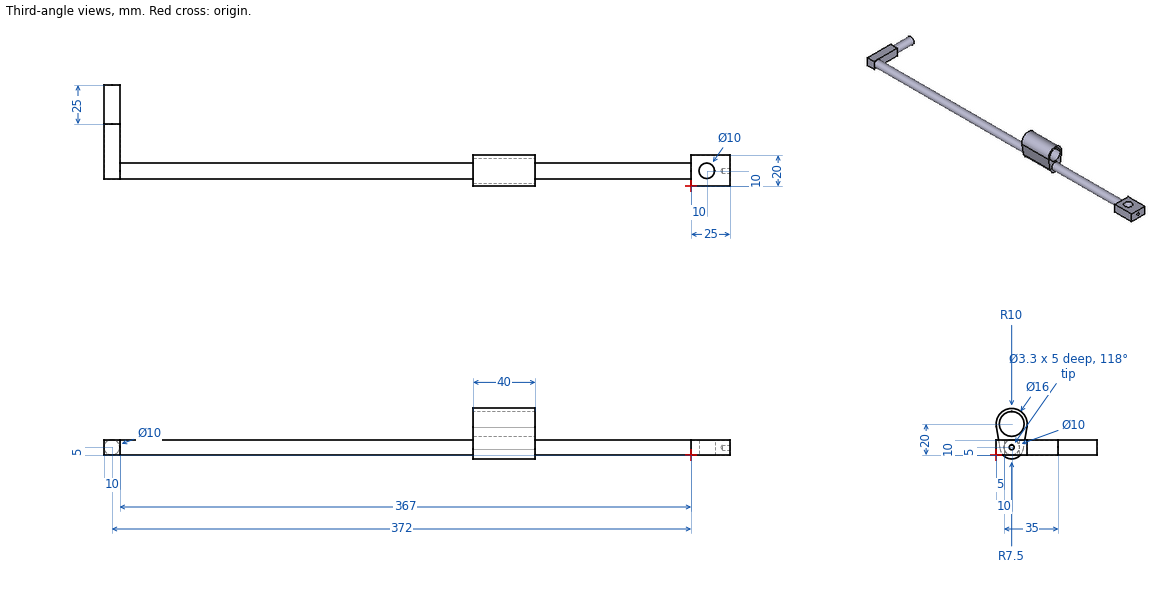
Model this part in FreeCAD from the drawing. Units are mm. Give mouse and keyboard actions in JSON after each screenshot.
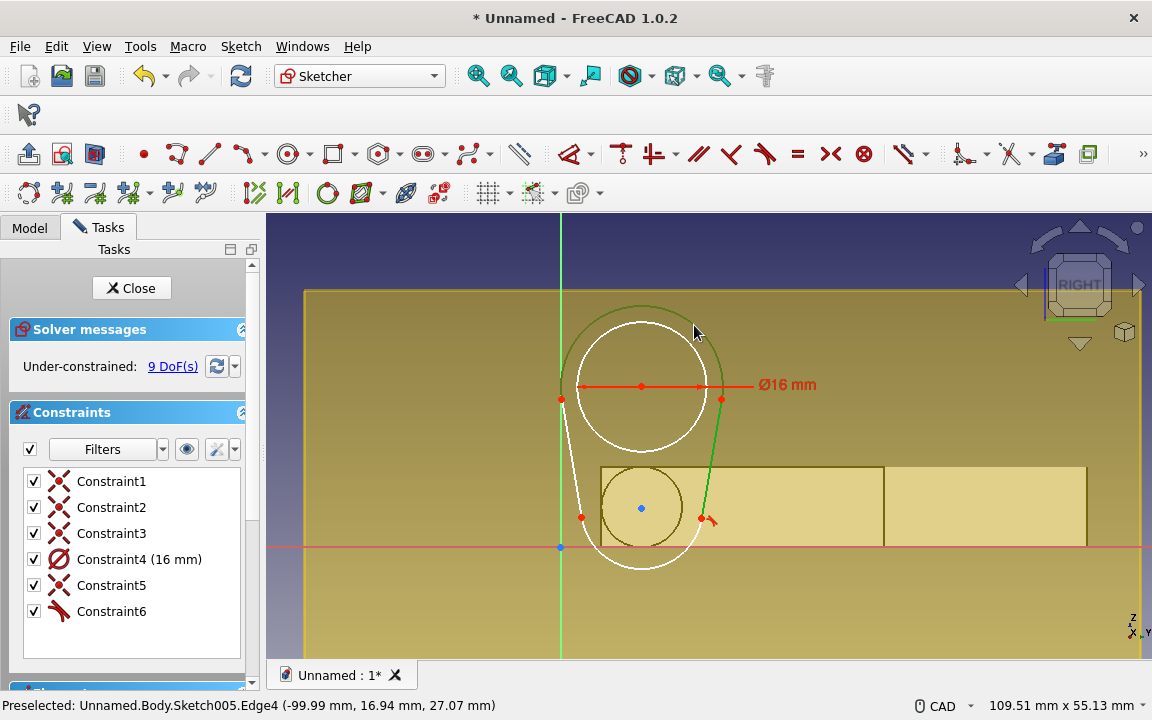
{"action": "key", "text": "t"}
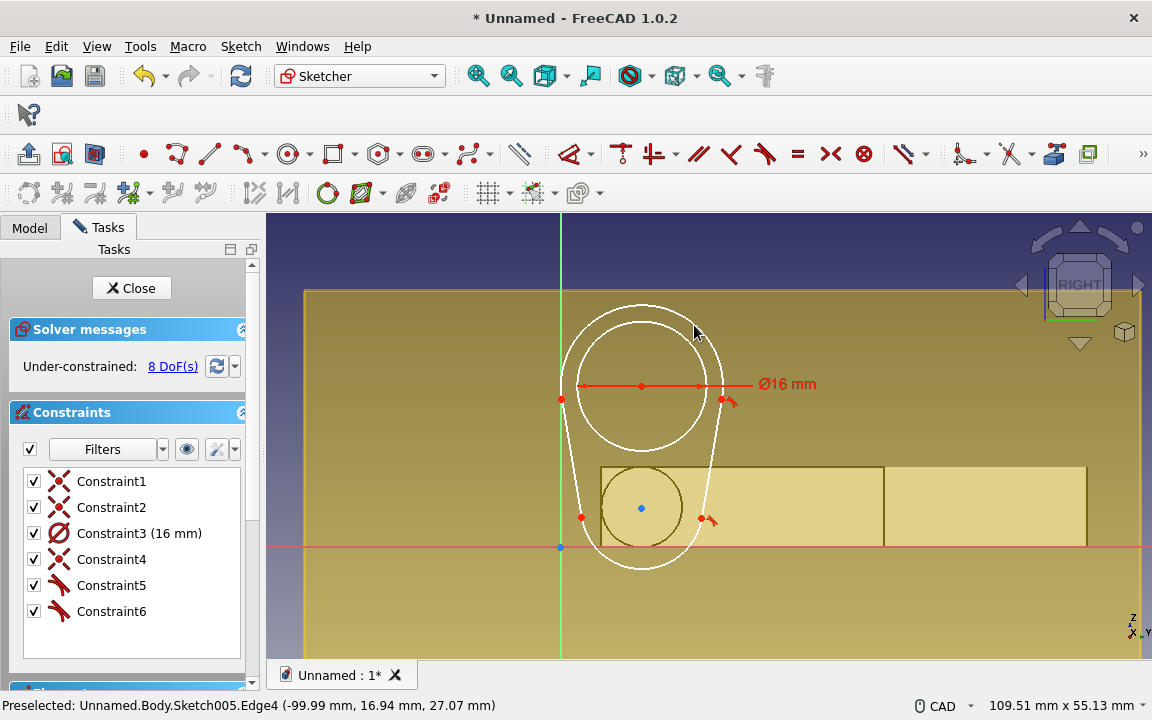
{"action": "left_click", "coordinate": [576, 482]}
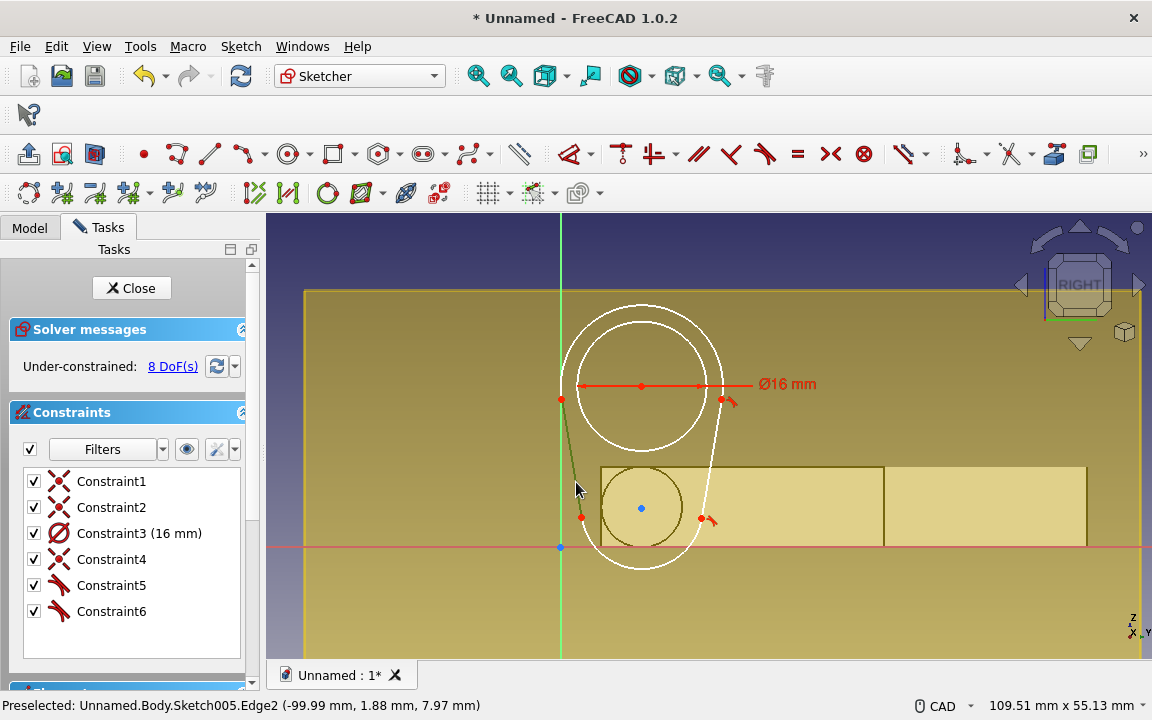
{"action": "left_click", "coordinate": [609, 559]}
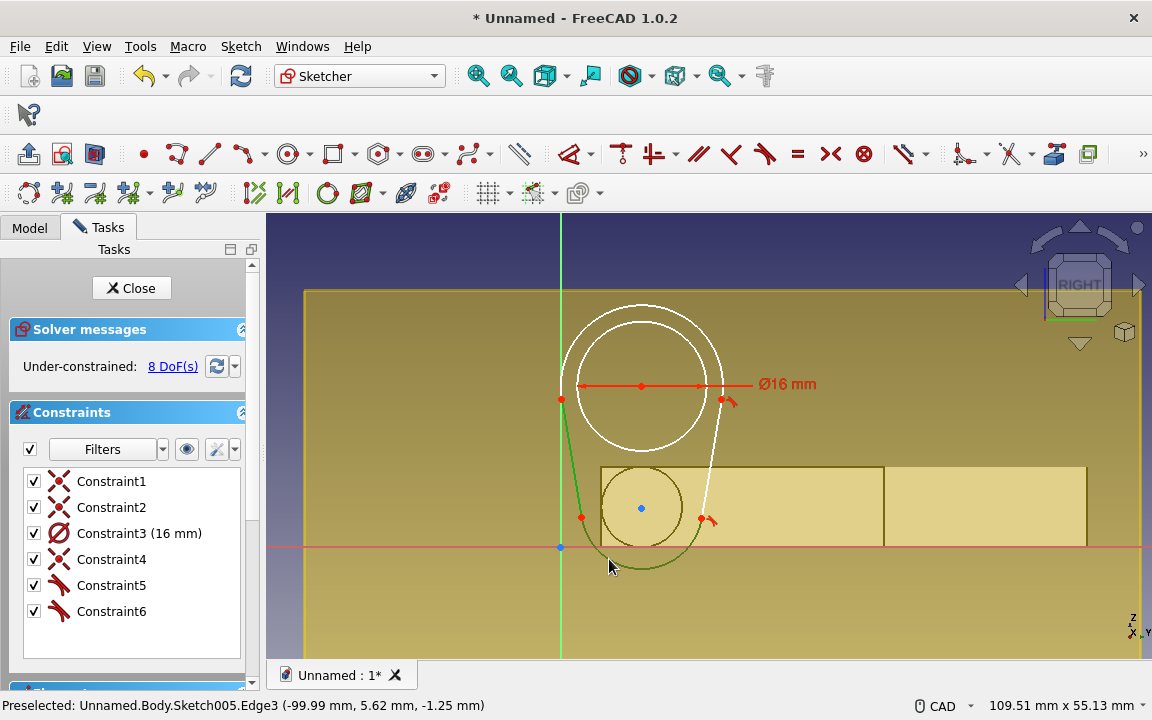
{"action": "key", "text": "t"}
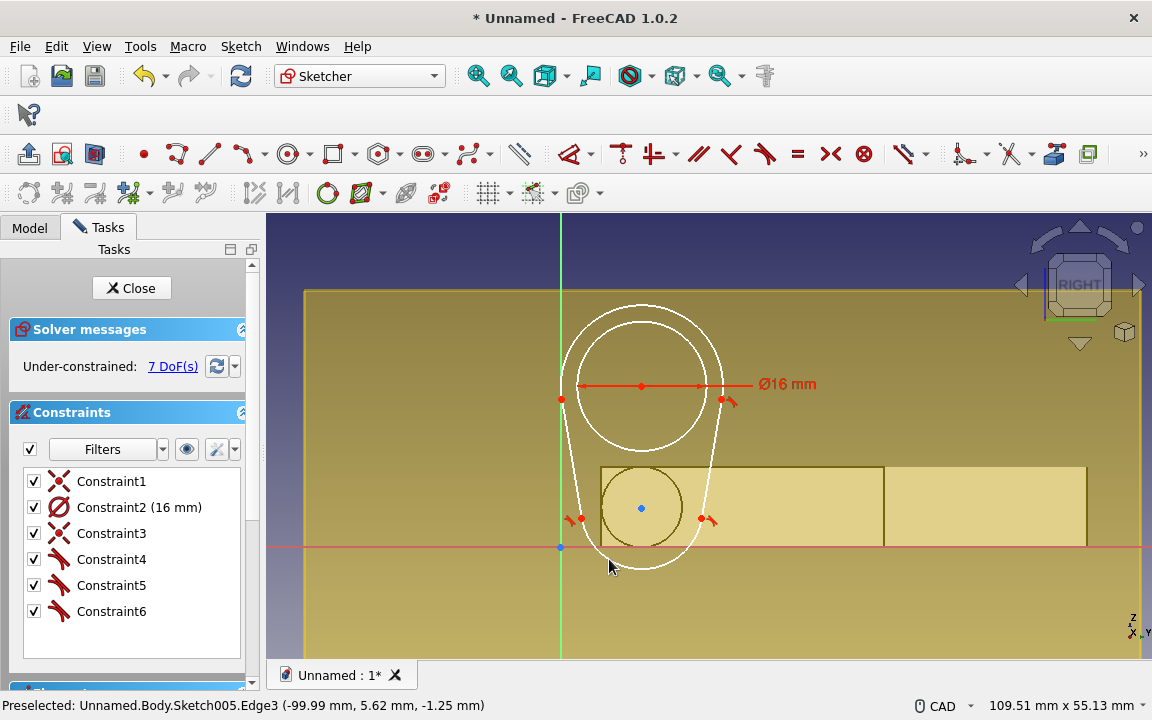
{"action": "left_click", "coordinate": [576, 483]}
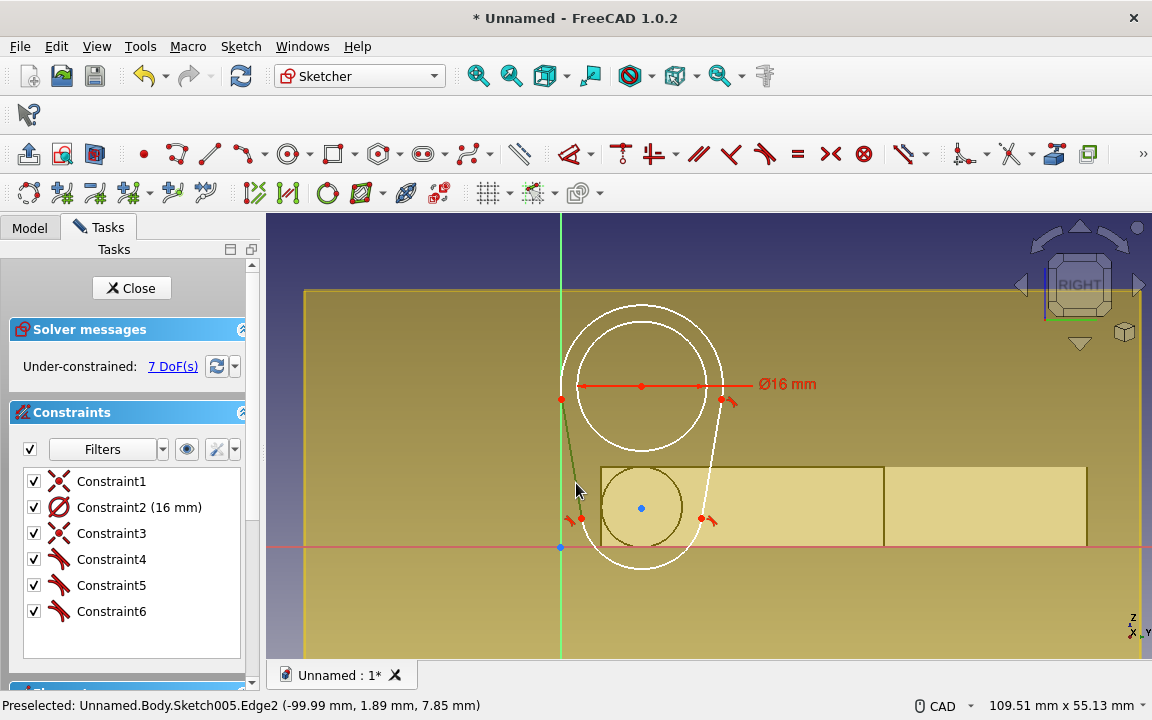
{"action": "left_click", "coordinate": [694, 324]}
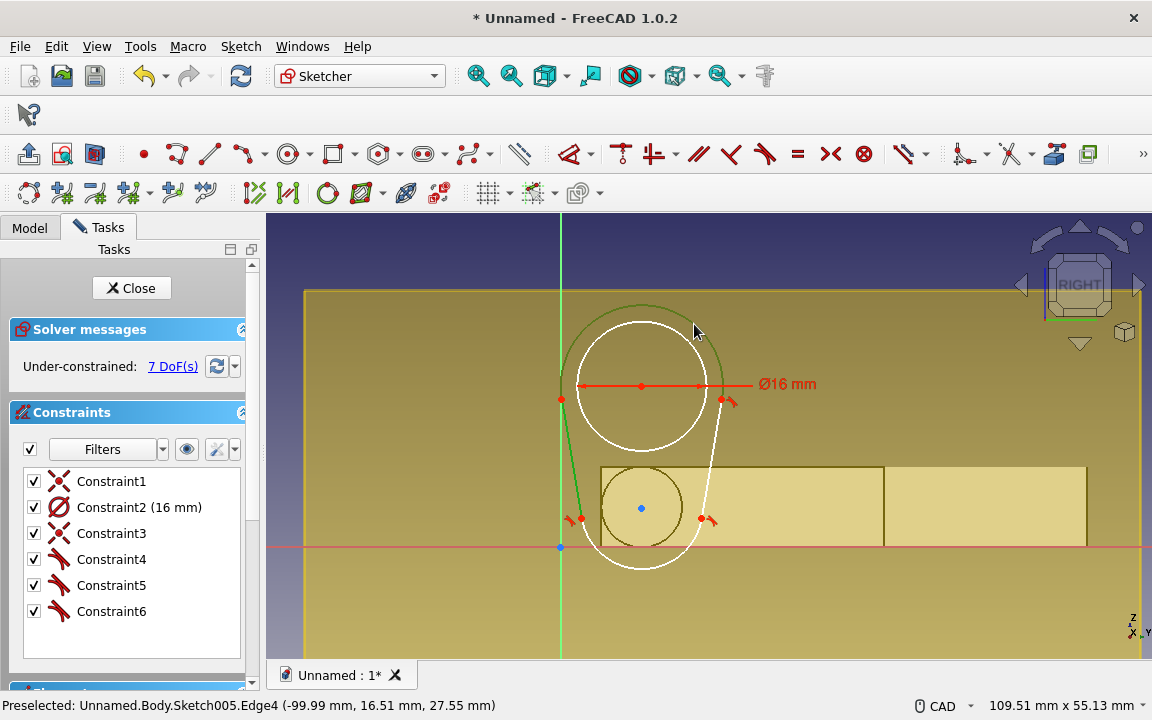
{"action": "key", "text": "t"}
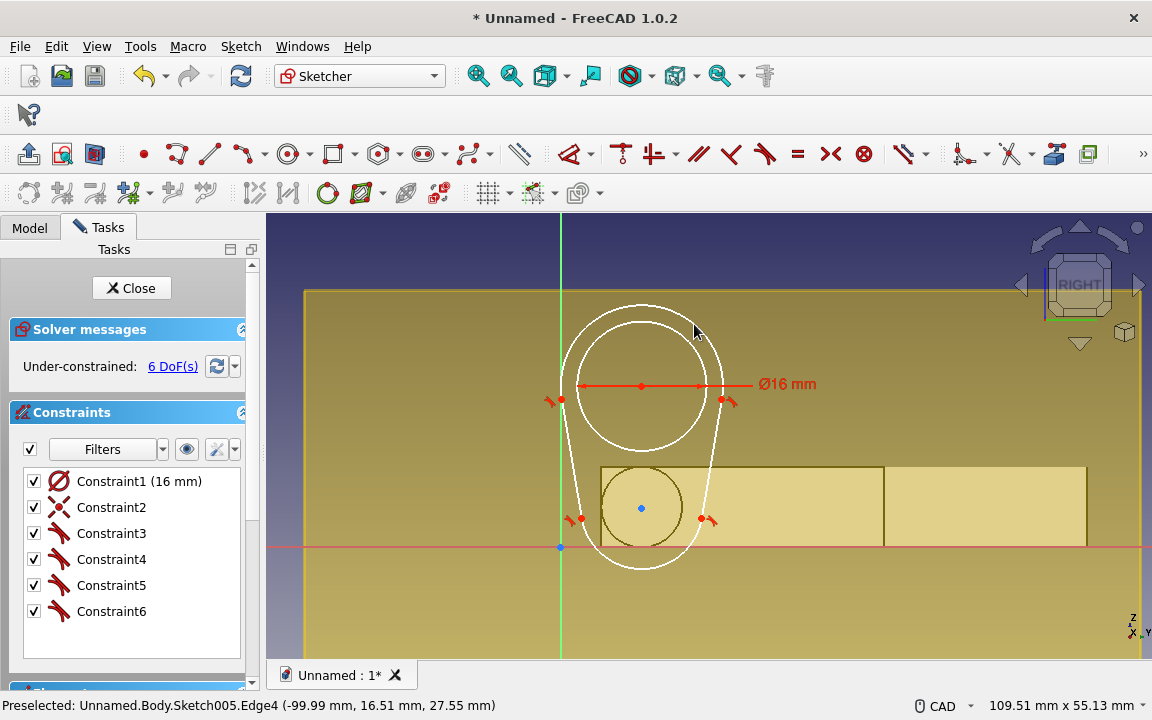
{"action": "key", "text": "d"}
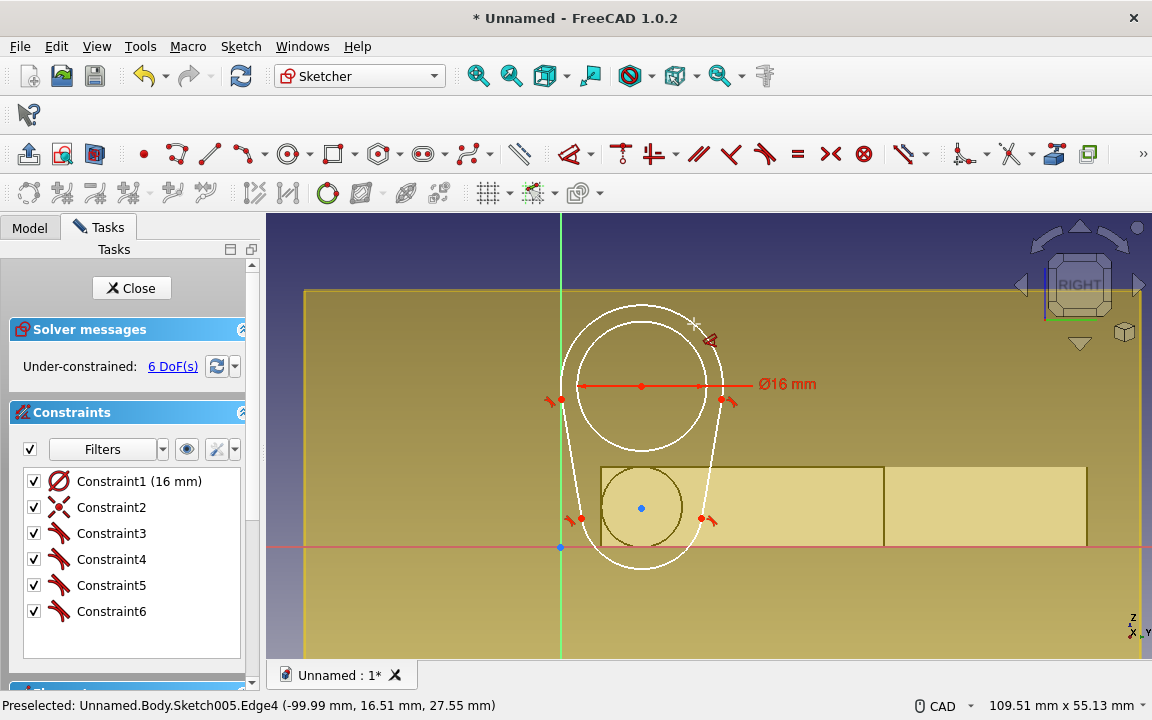
{"action": "left_click", "coordinate": [609, 560]}
{"action": "left_click", "coordinate": [592, 587]}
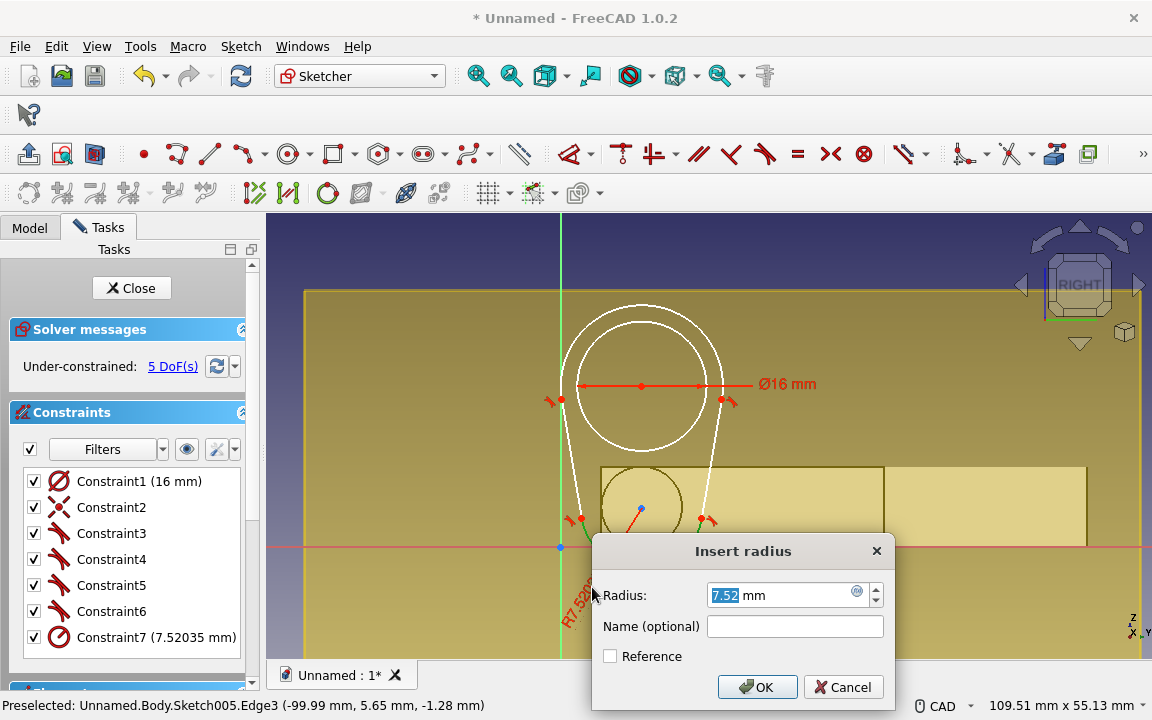
{"action": "type", "text": "7.5"}
{"action": "key", "text": "Return"}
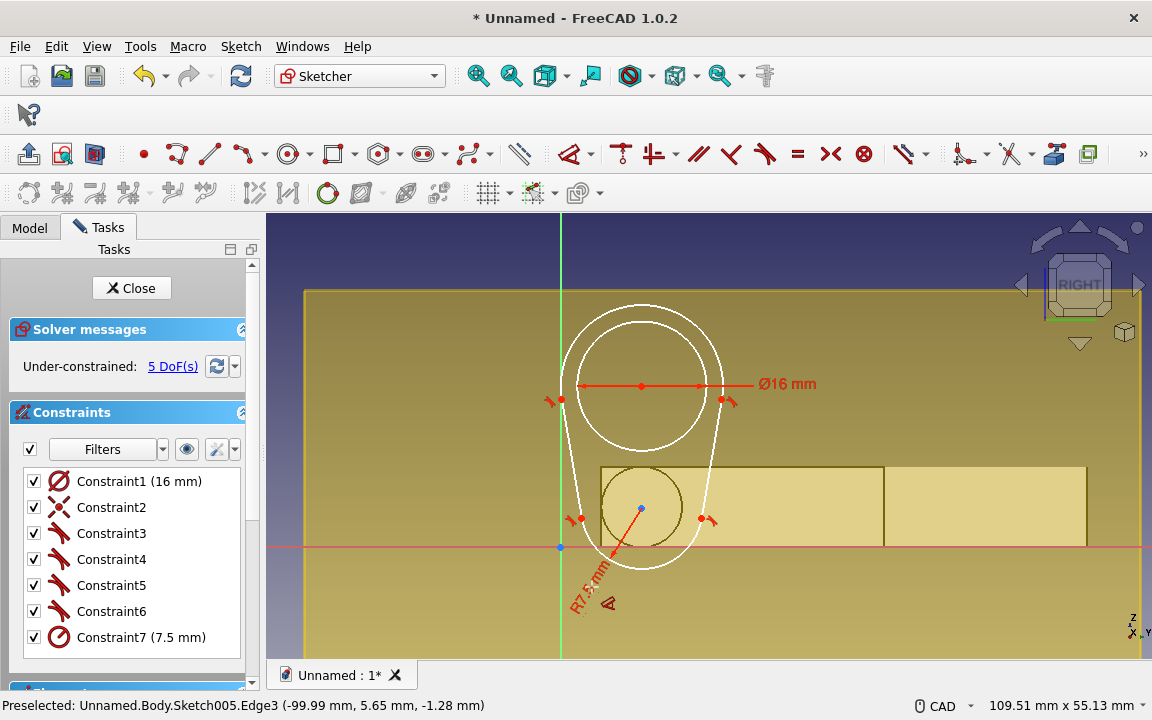
{"action": "left_click", "coordinate": [694, 324]}
{"action": "left_click", "coordinate": [715, 299]}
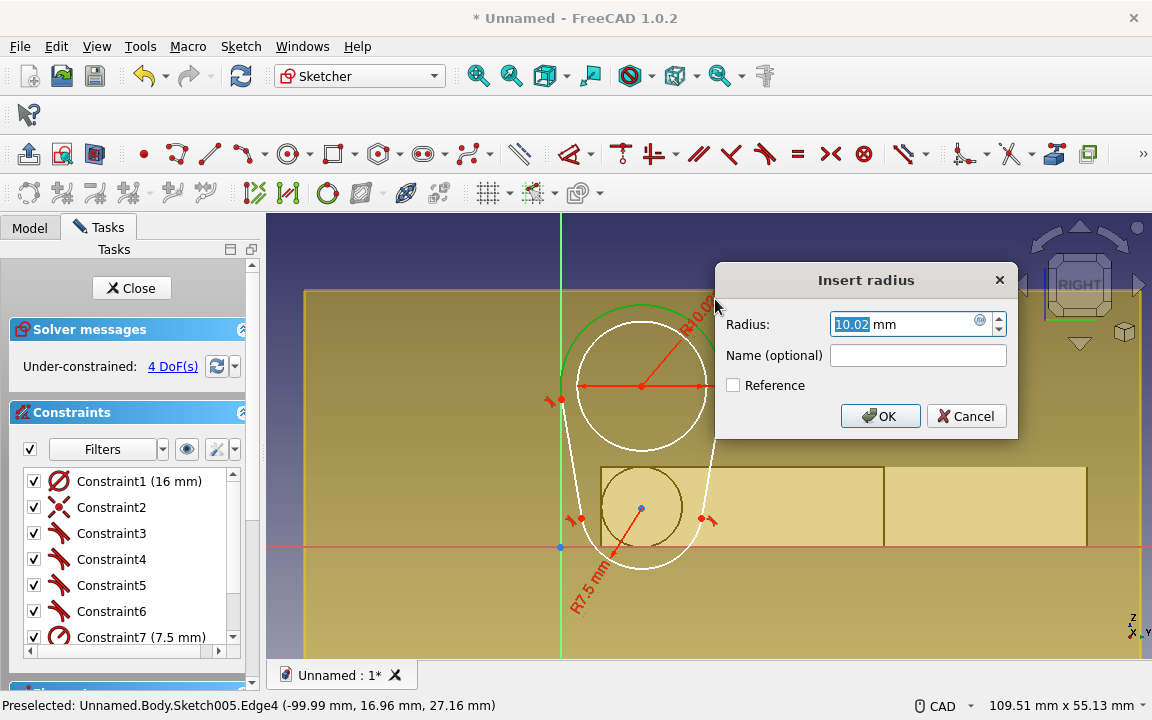
{"action": "type", "text": "10"}
{"action": "key", "text": "Return"}